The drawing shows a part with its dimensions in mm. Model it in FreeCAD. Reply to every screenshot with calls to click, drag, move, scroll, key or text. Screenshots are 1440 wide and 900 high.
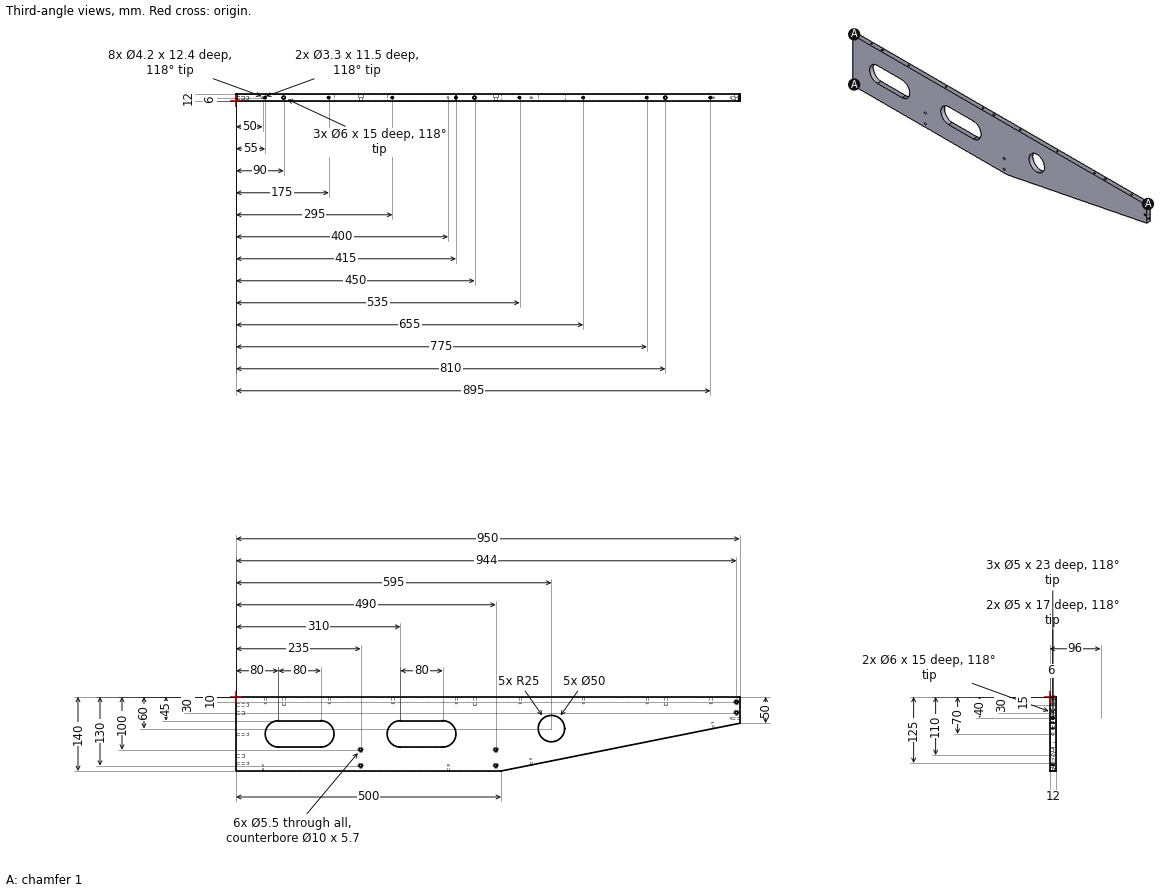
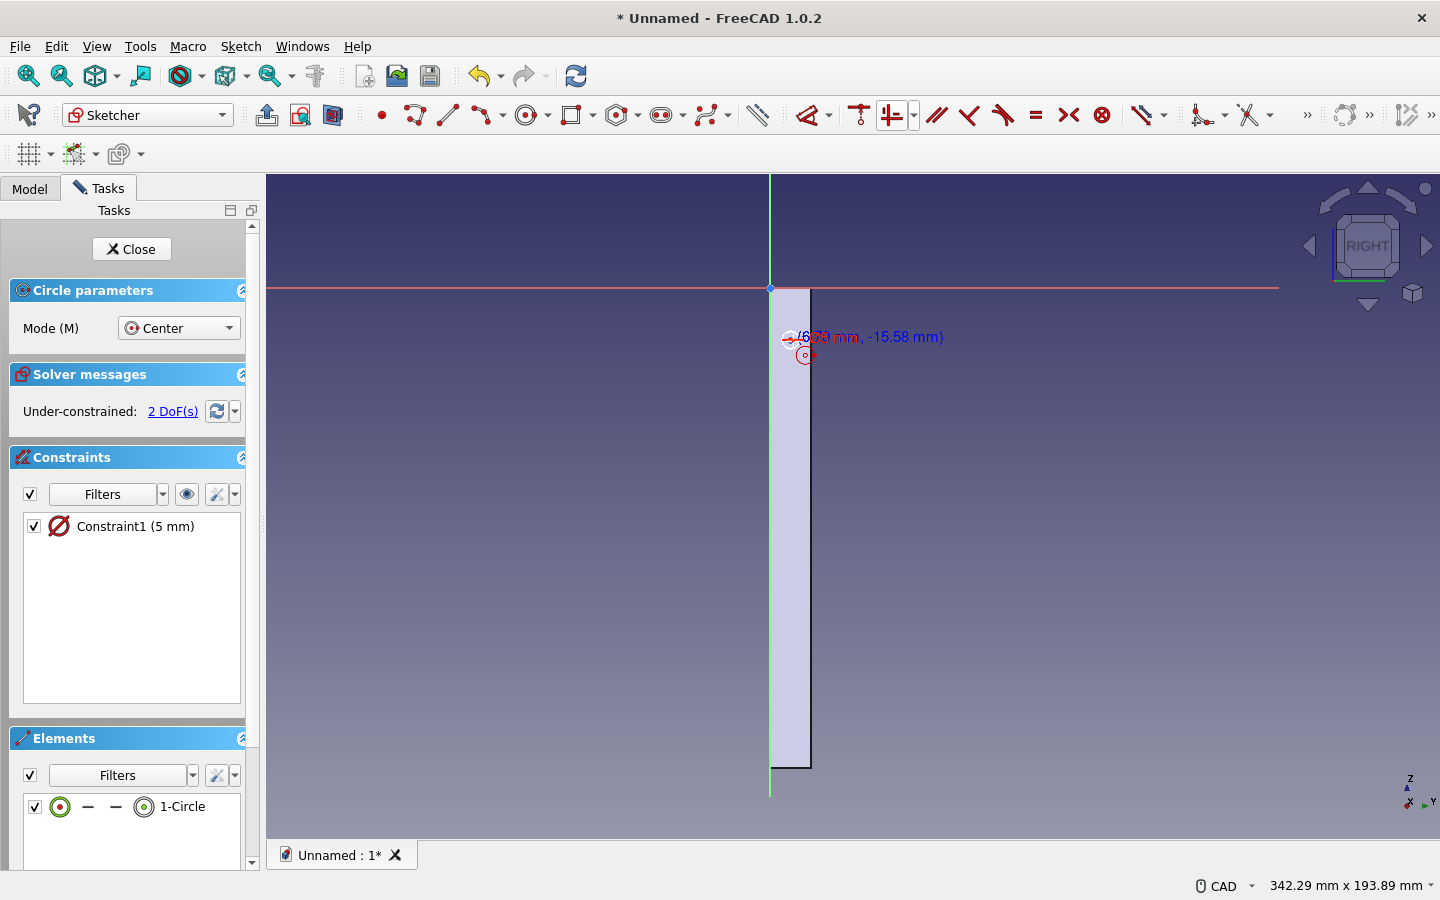
scroll(791, 528, up, 5)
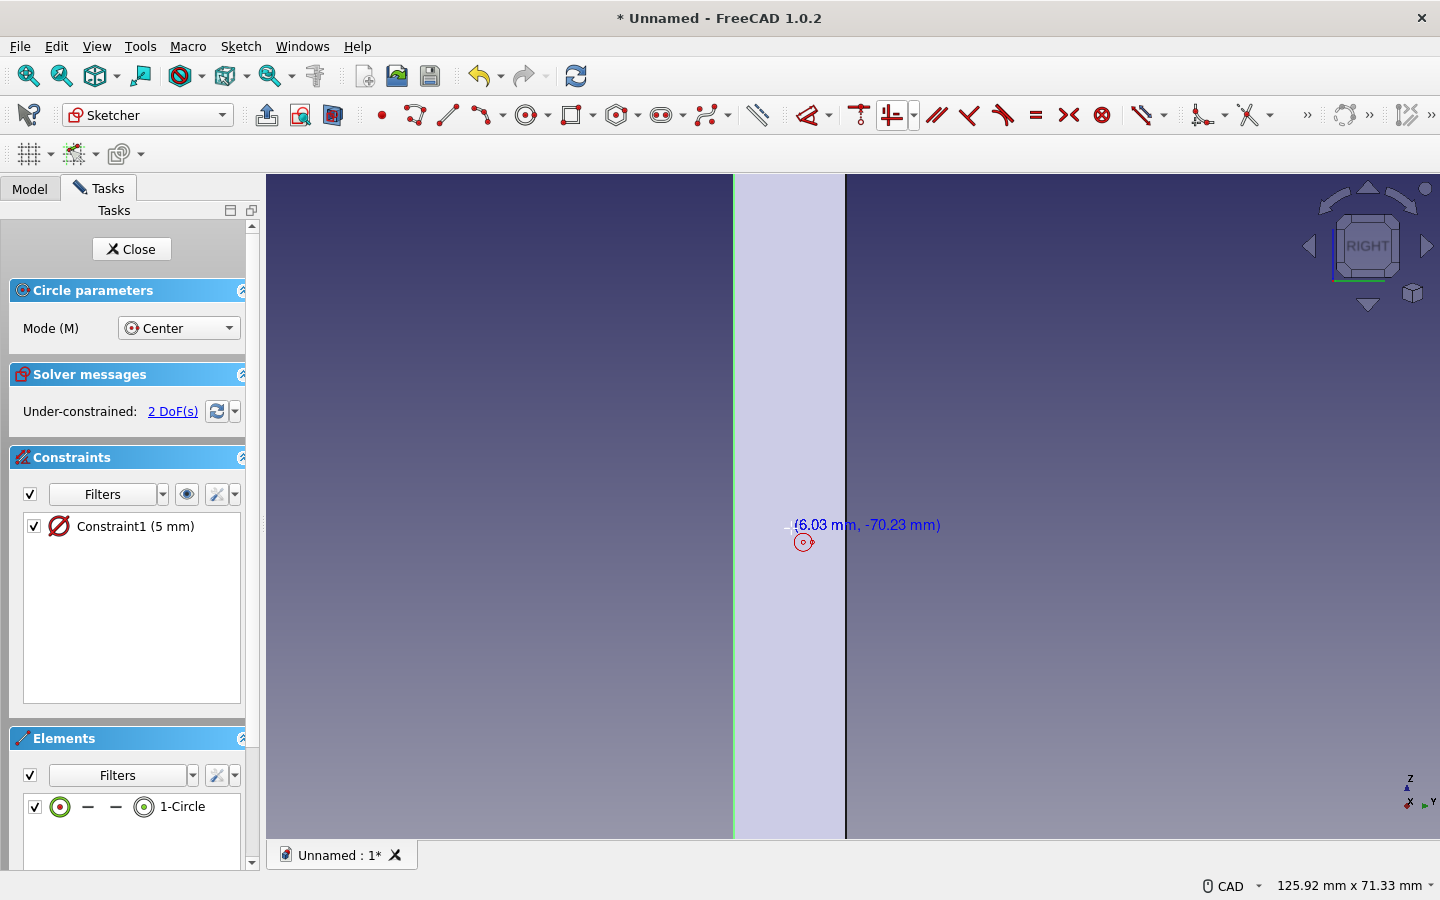
click(790, 528)
move(806, 511)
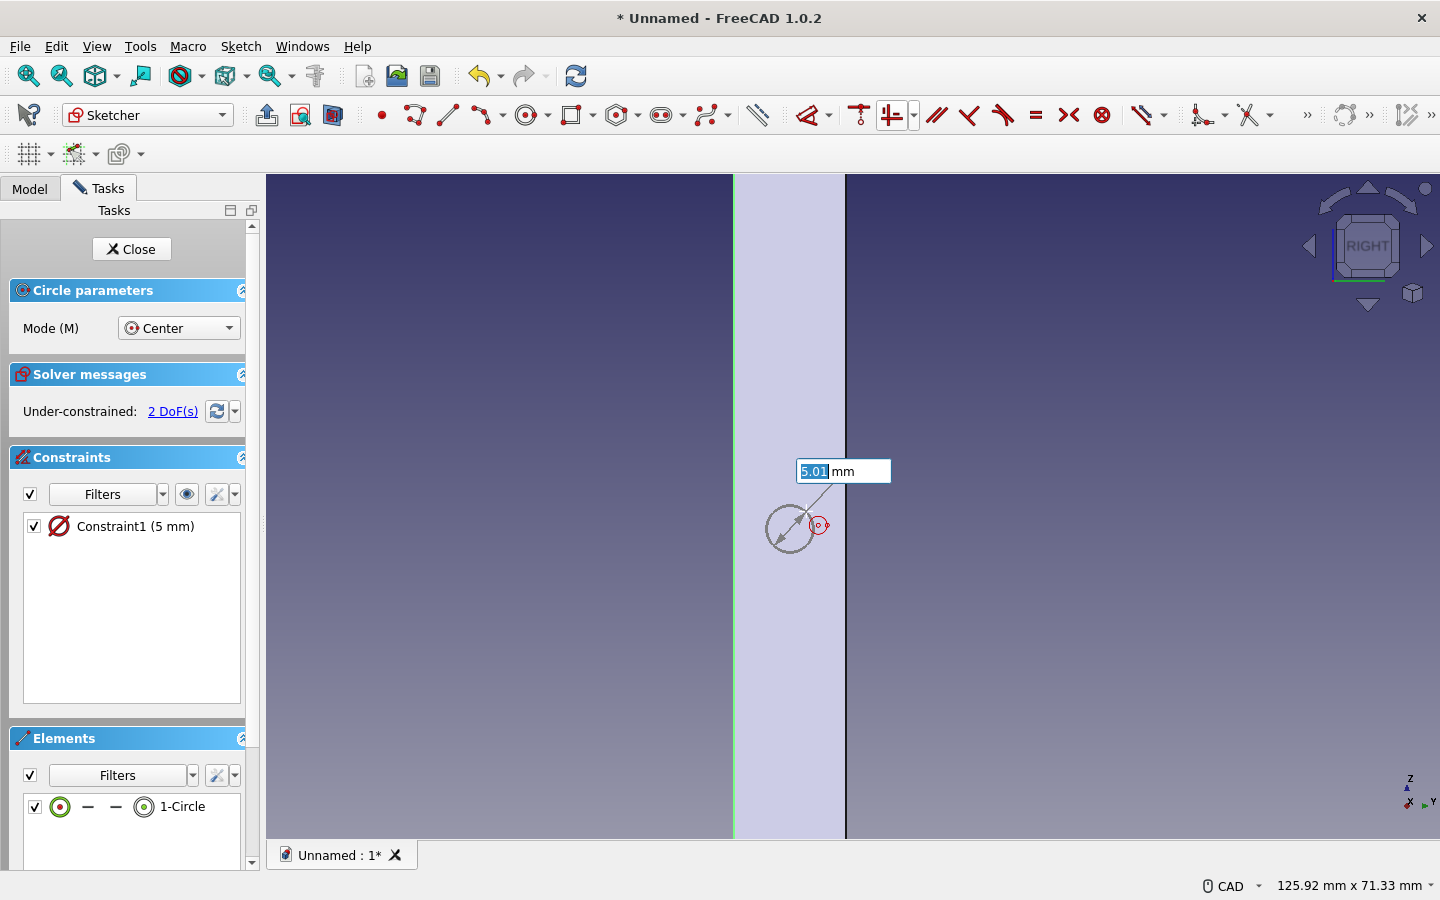
text(5)
key(Return)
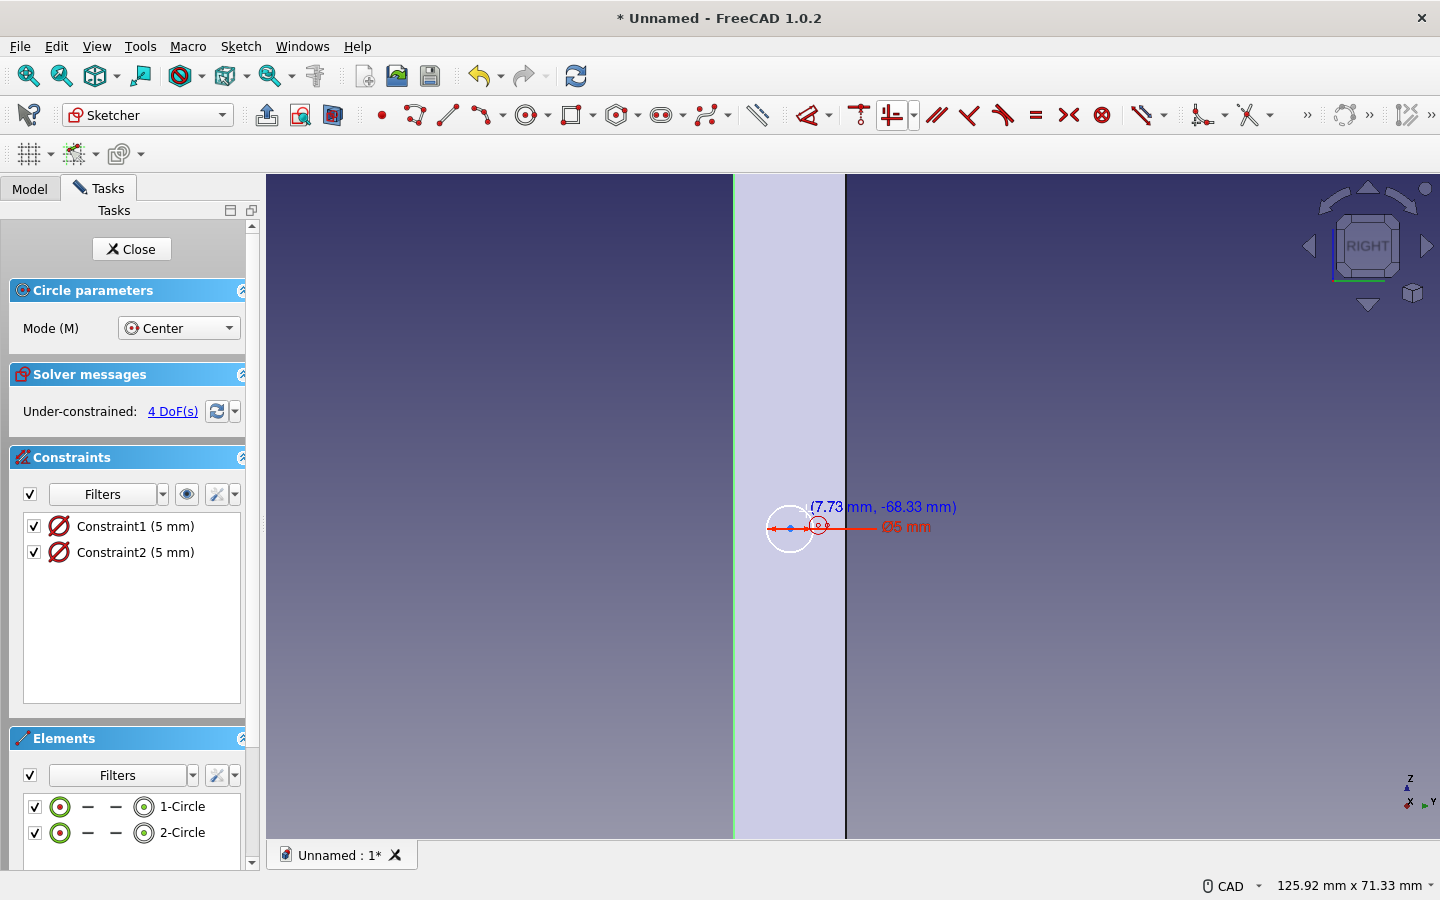
scroll(791, 528, down, 5)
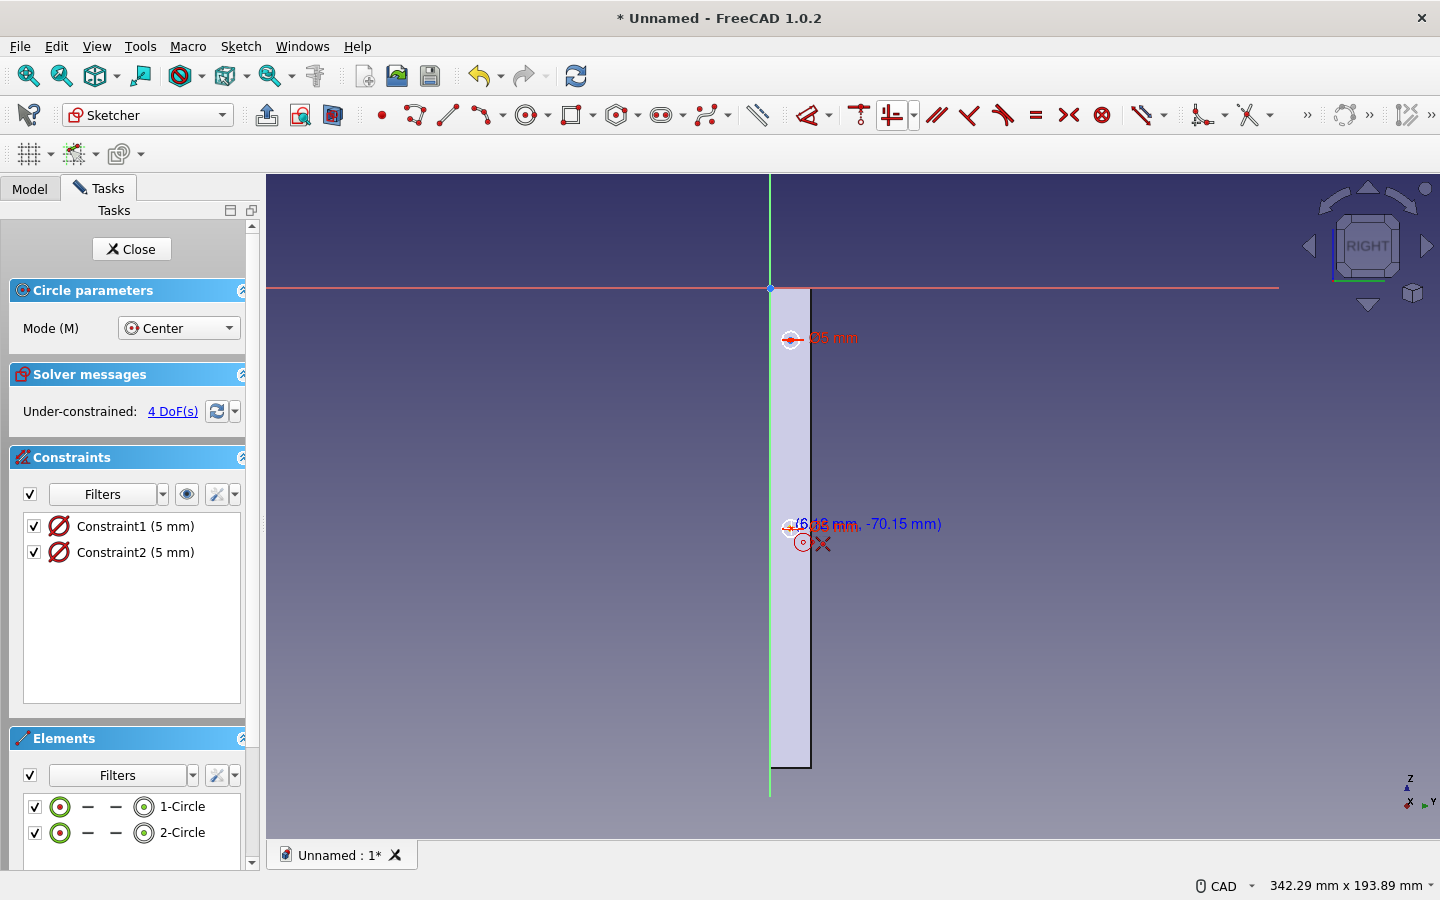
scroll(791, 717, up, 5)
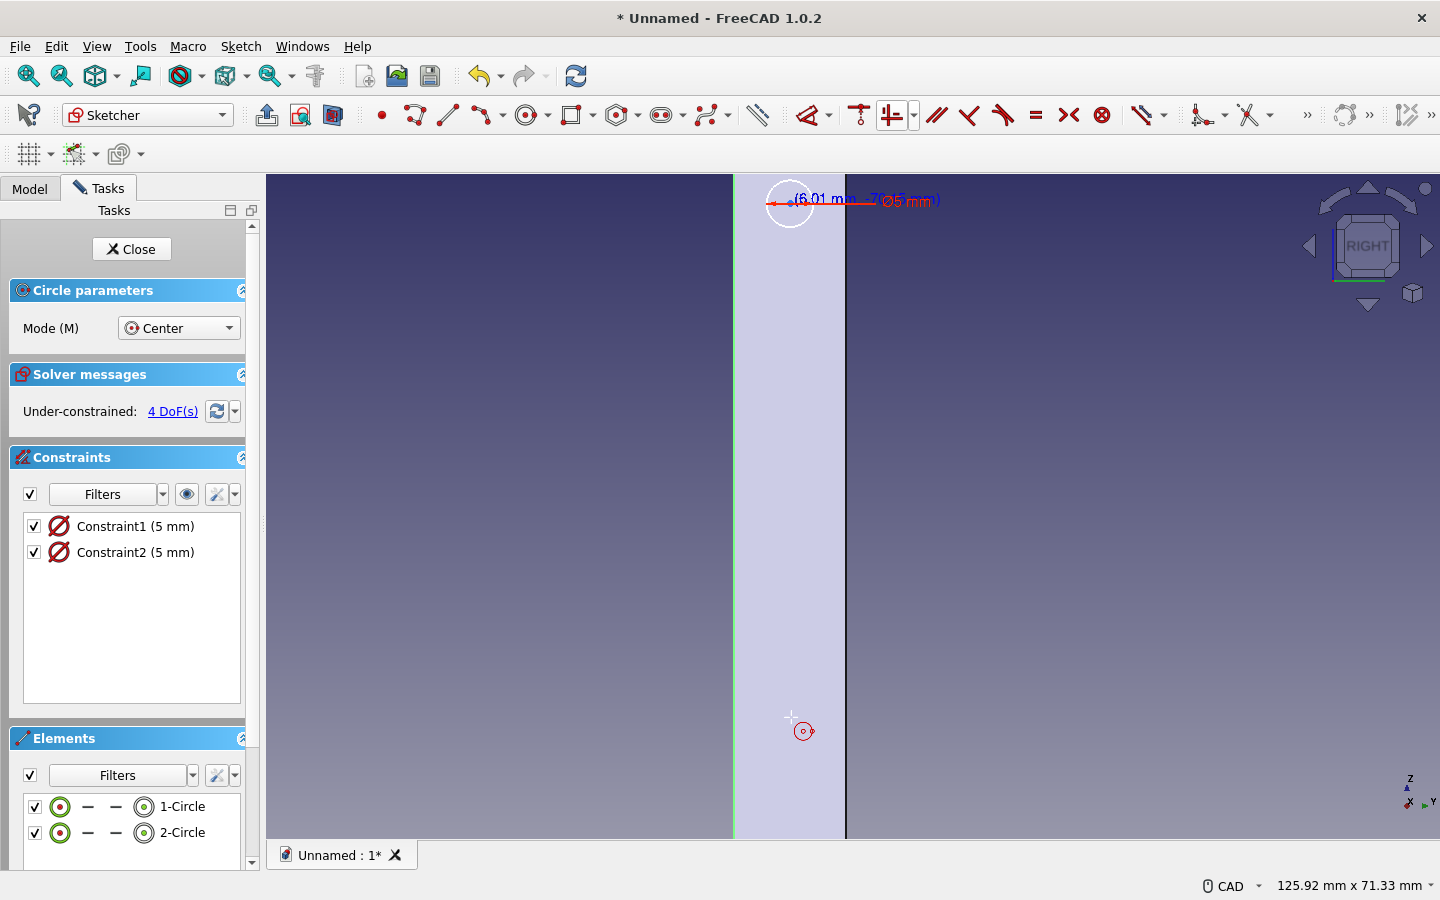
click(790, 715)
move(806, 699)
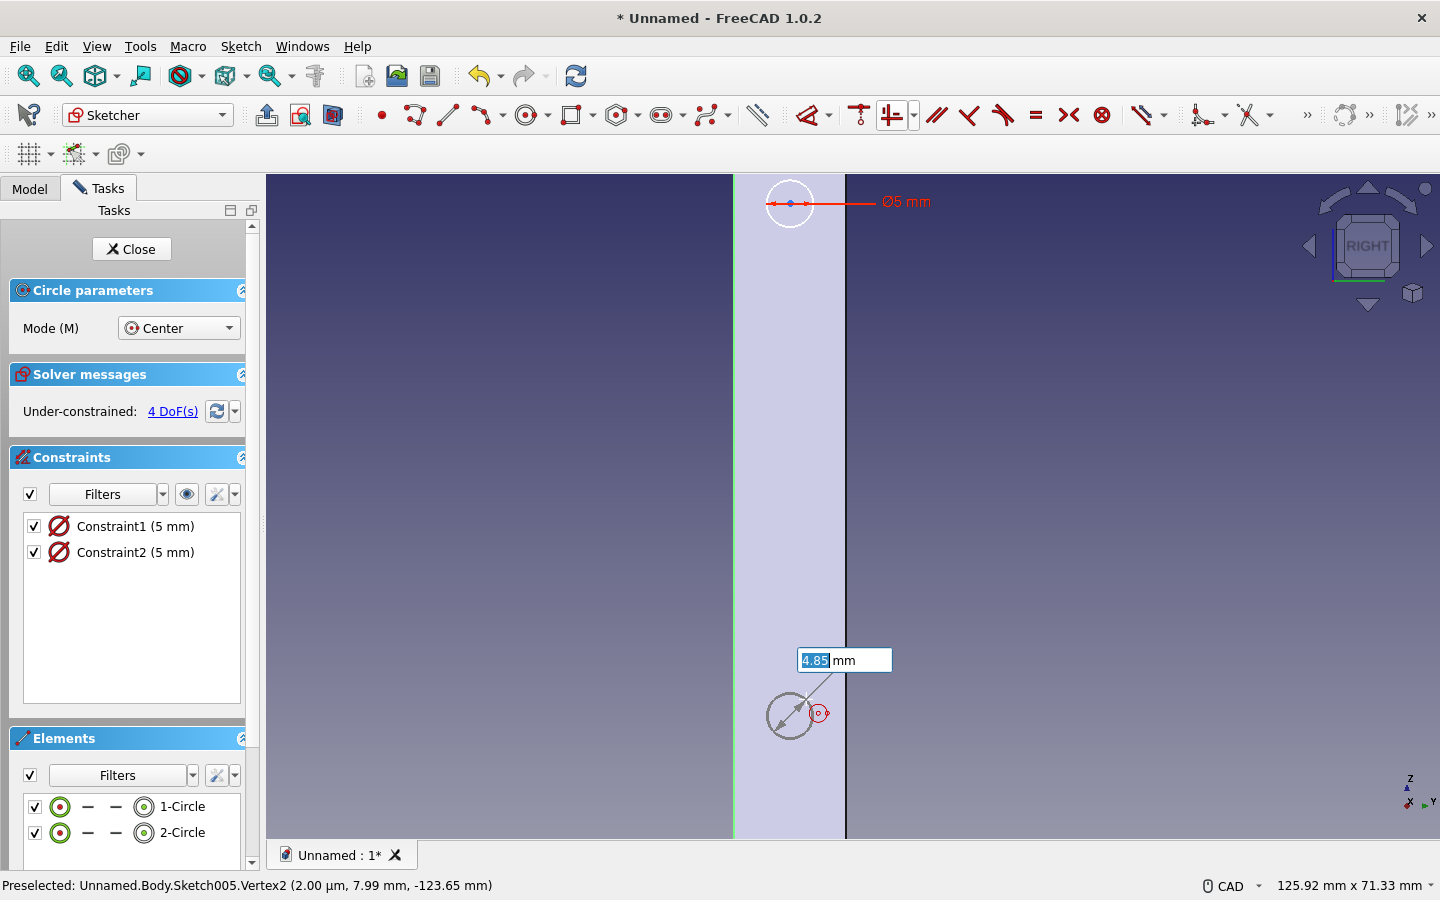
text(5)
key(Return)
key(Escape)